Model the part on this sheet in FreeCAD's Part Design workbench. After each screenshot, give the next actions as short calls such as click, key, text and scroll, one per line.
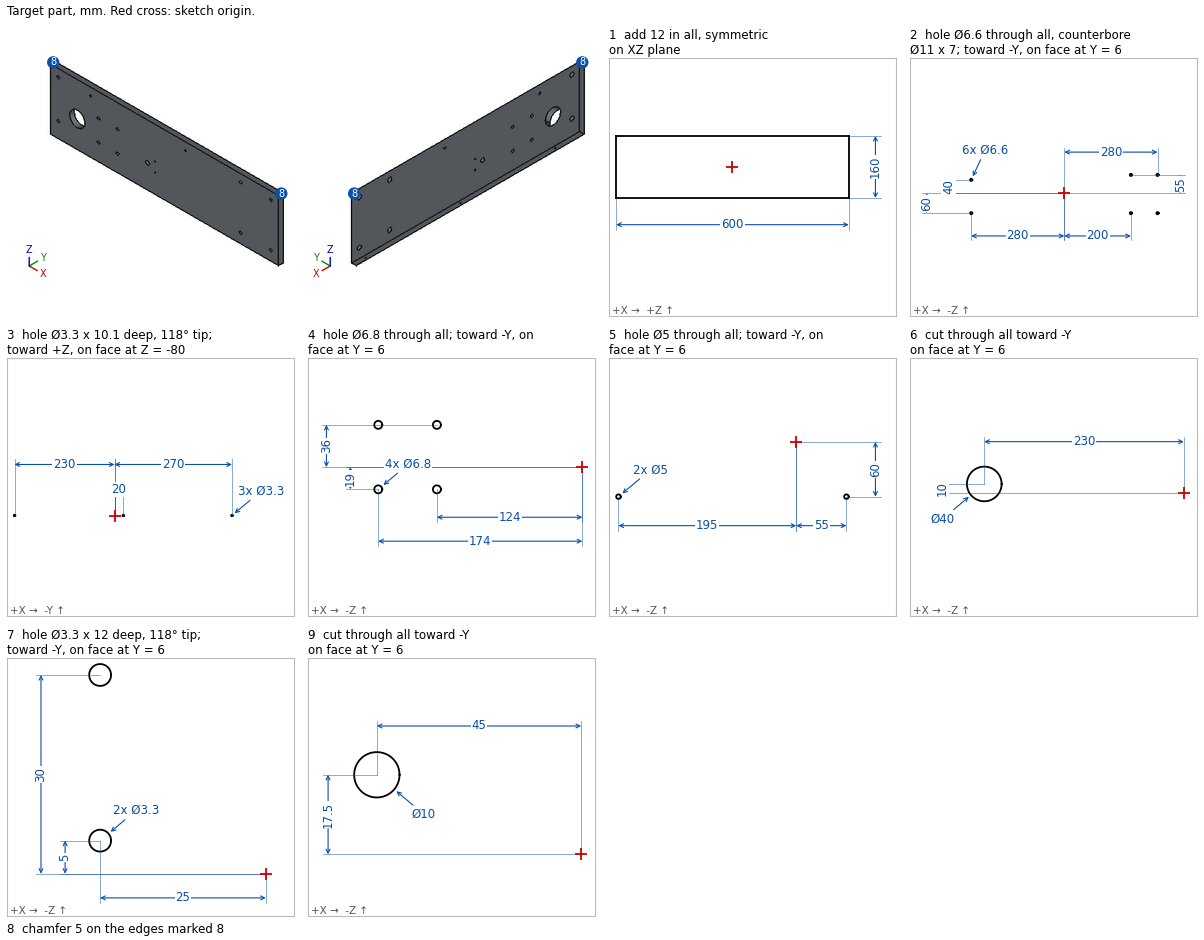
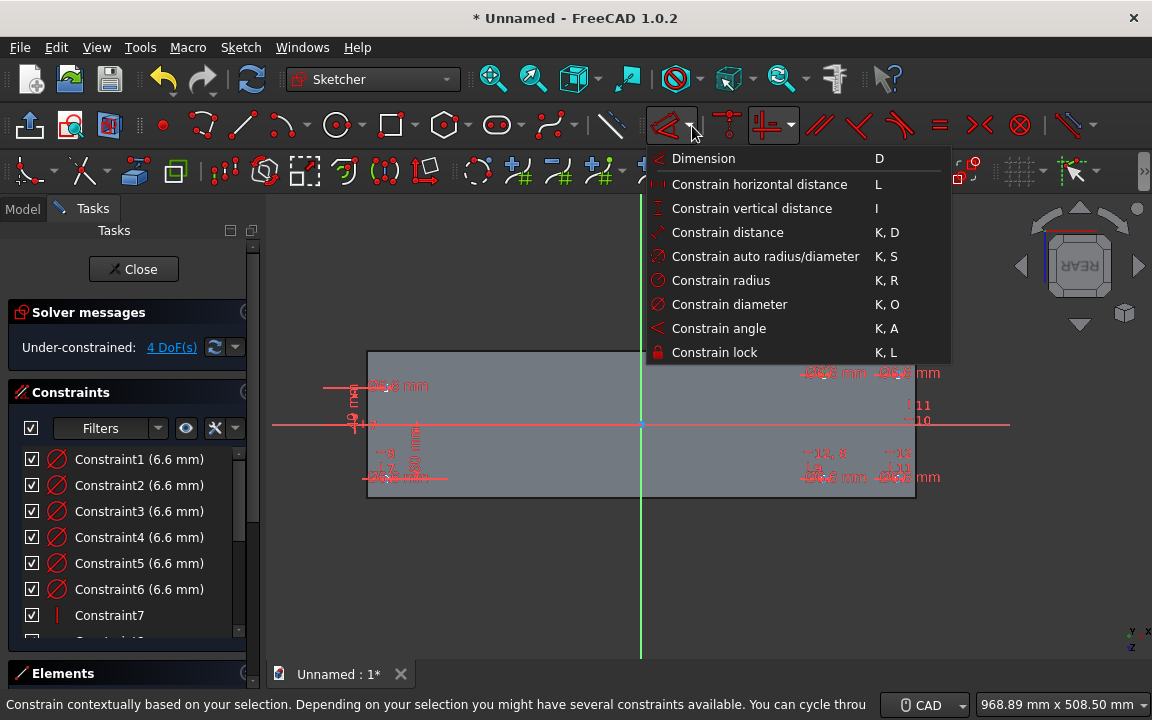
click(799, 208)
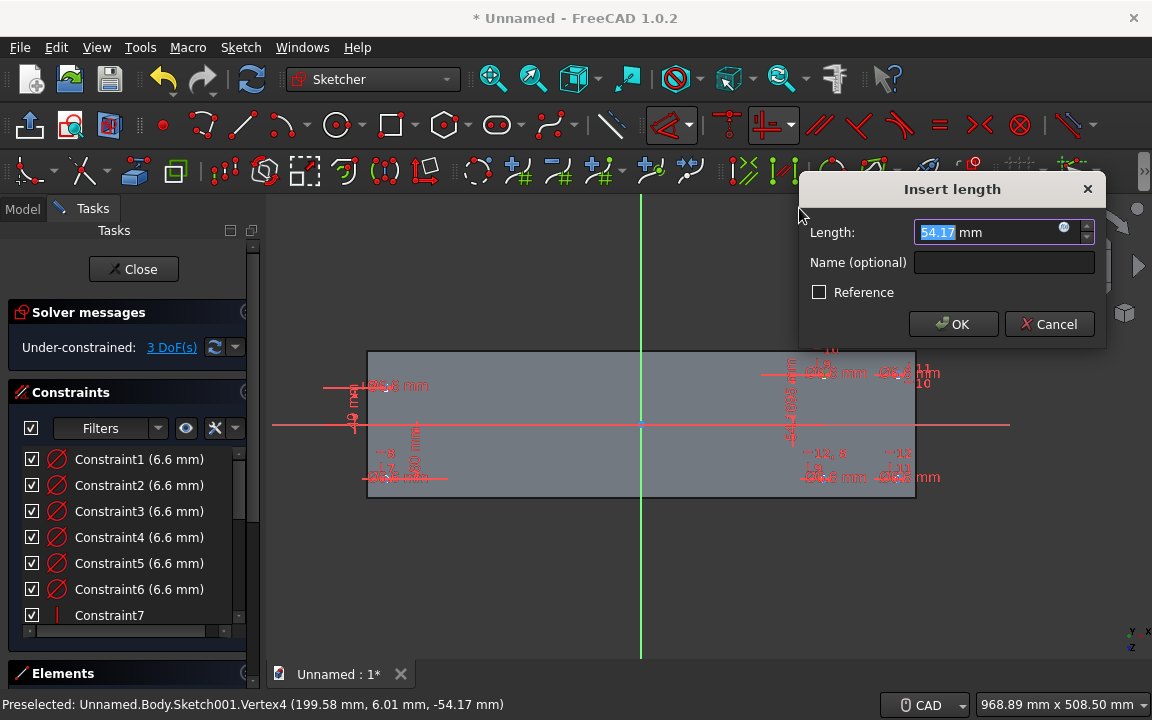
text(55)
key(Return)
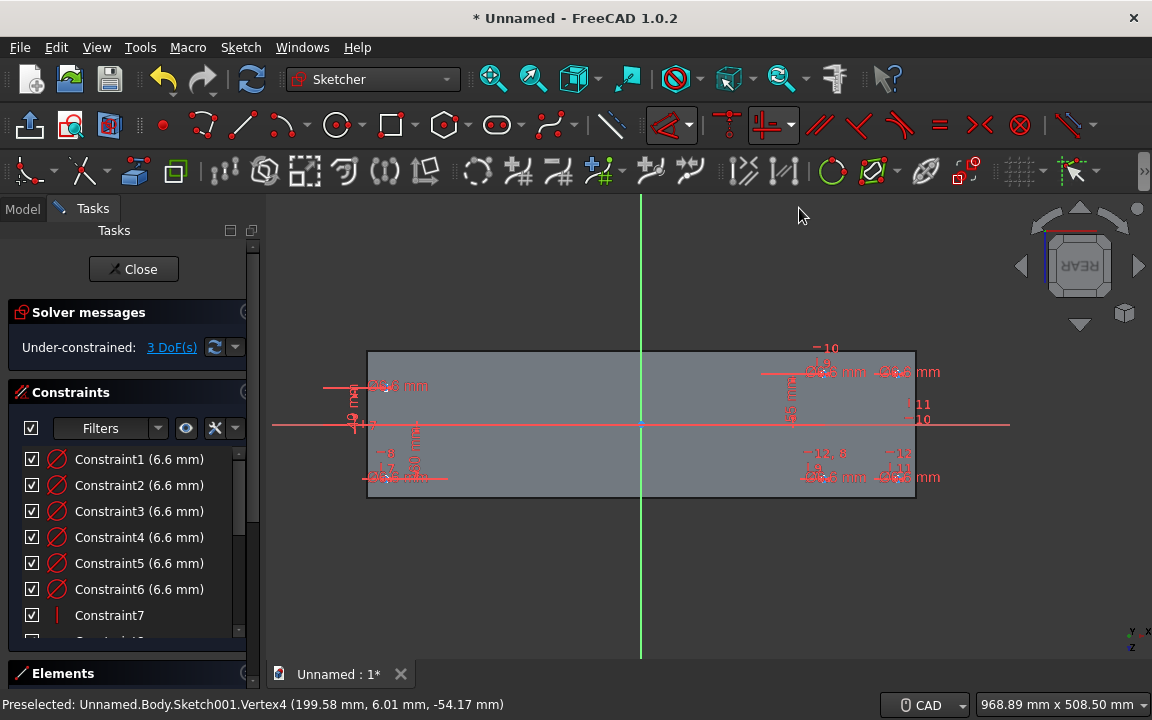
click(386, 479)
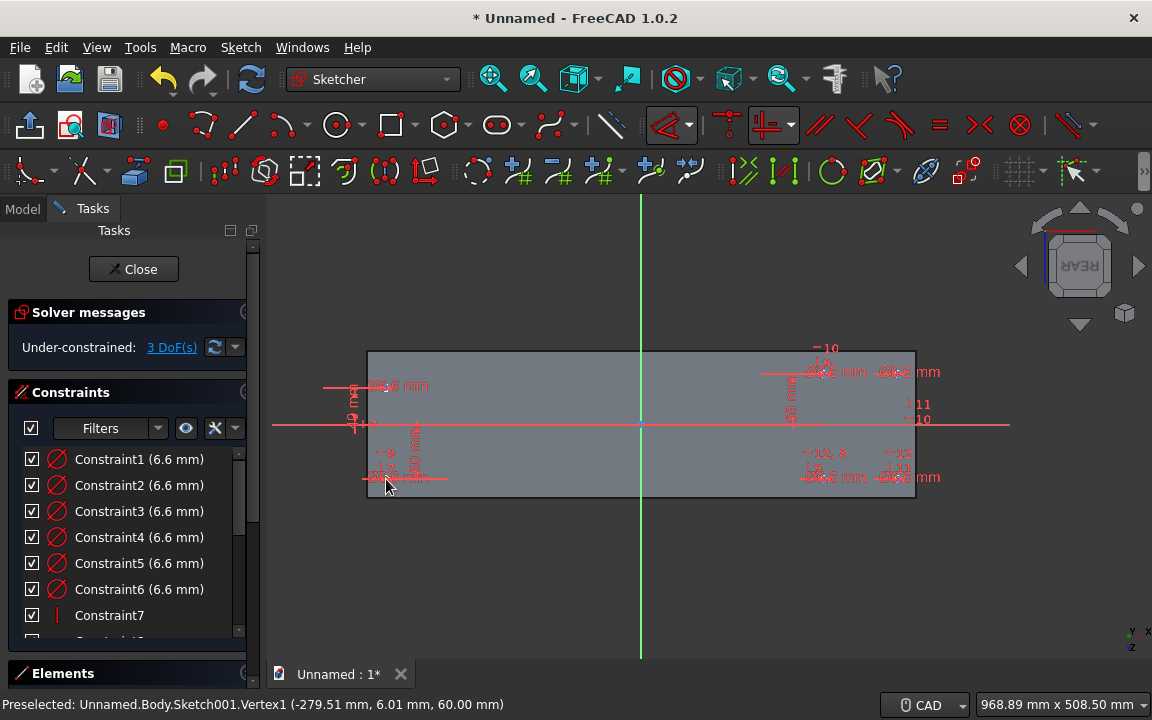
click(692, 126)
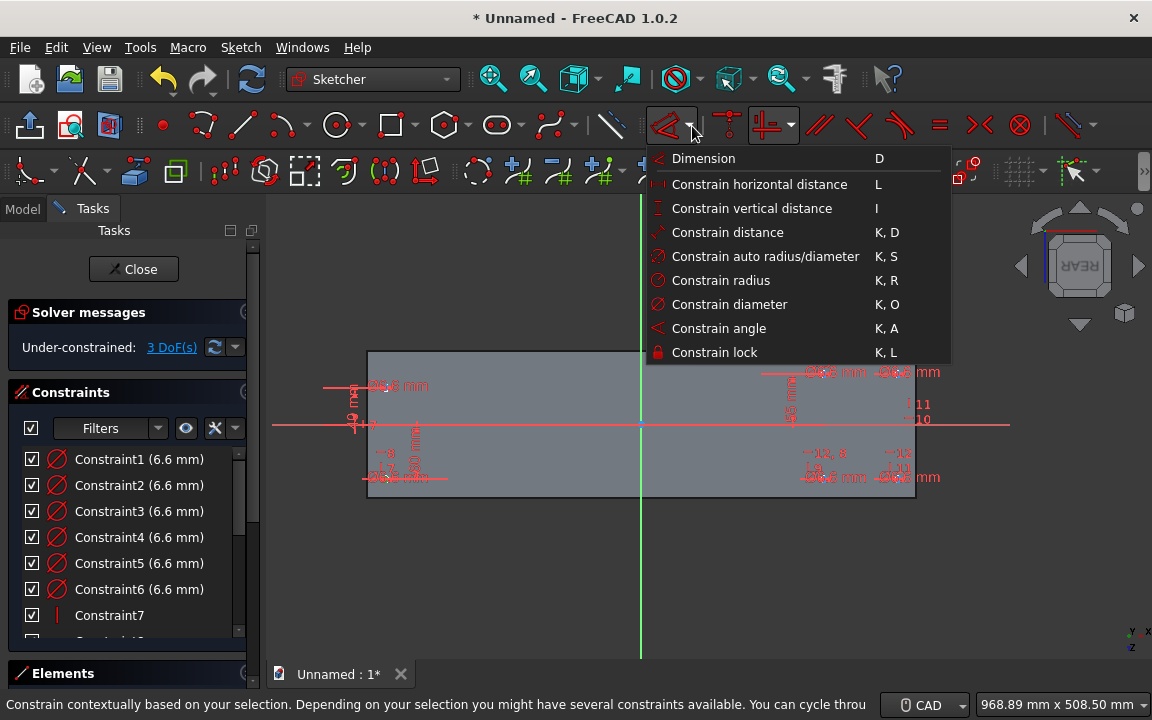
click(799, 184)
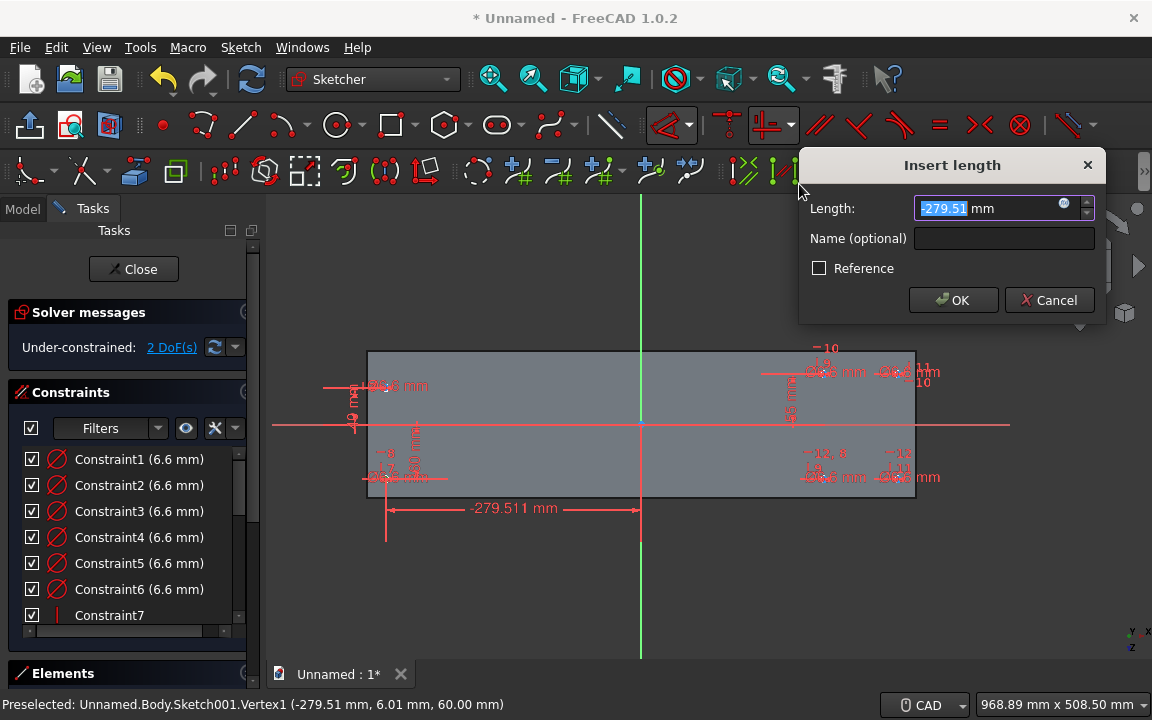
text(-280)
key(Return)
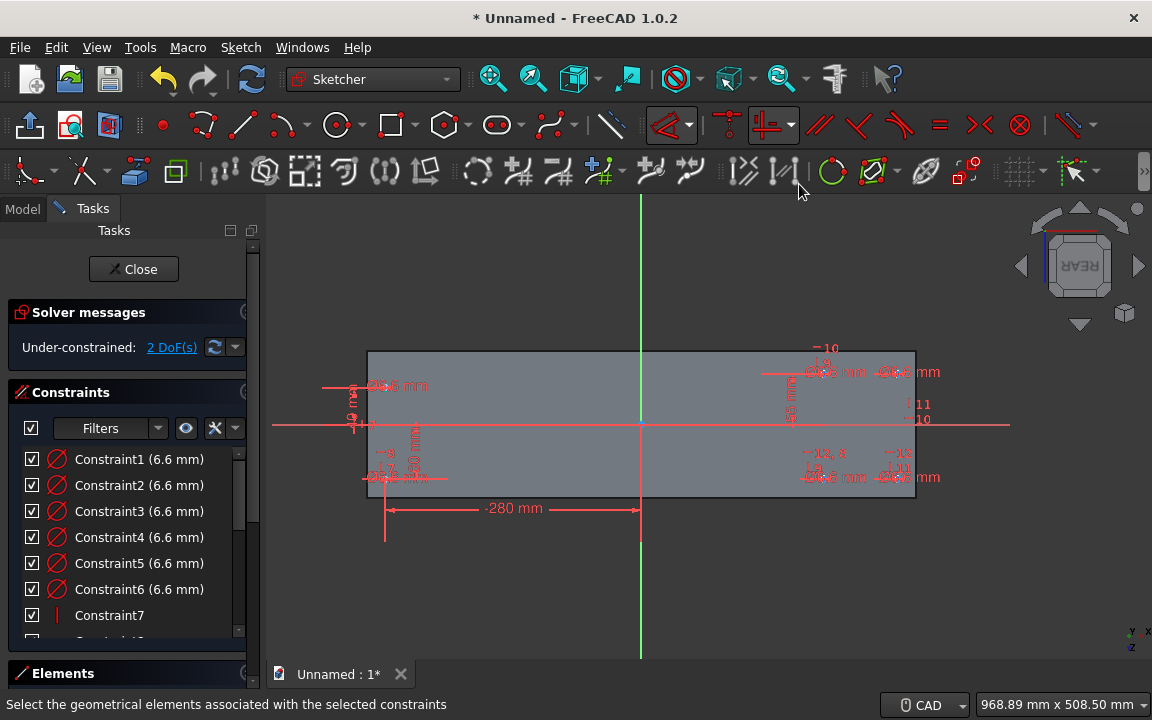
click(824, 479)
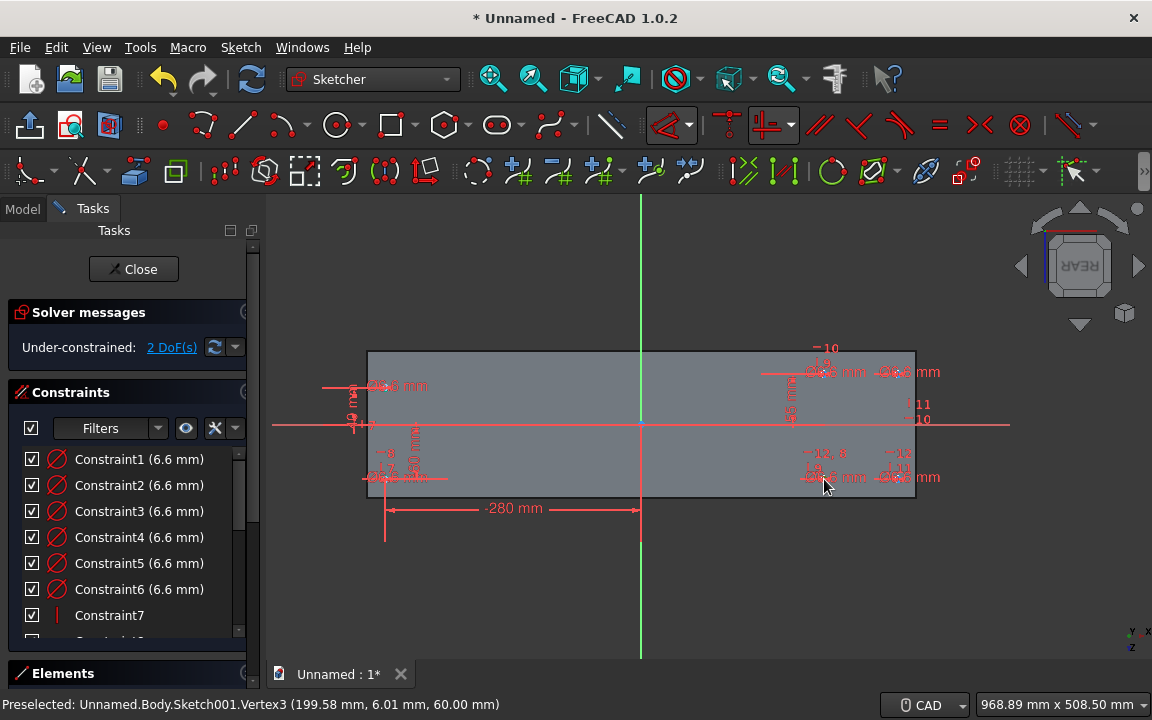
click(692, 126)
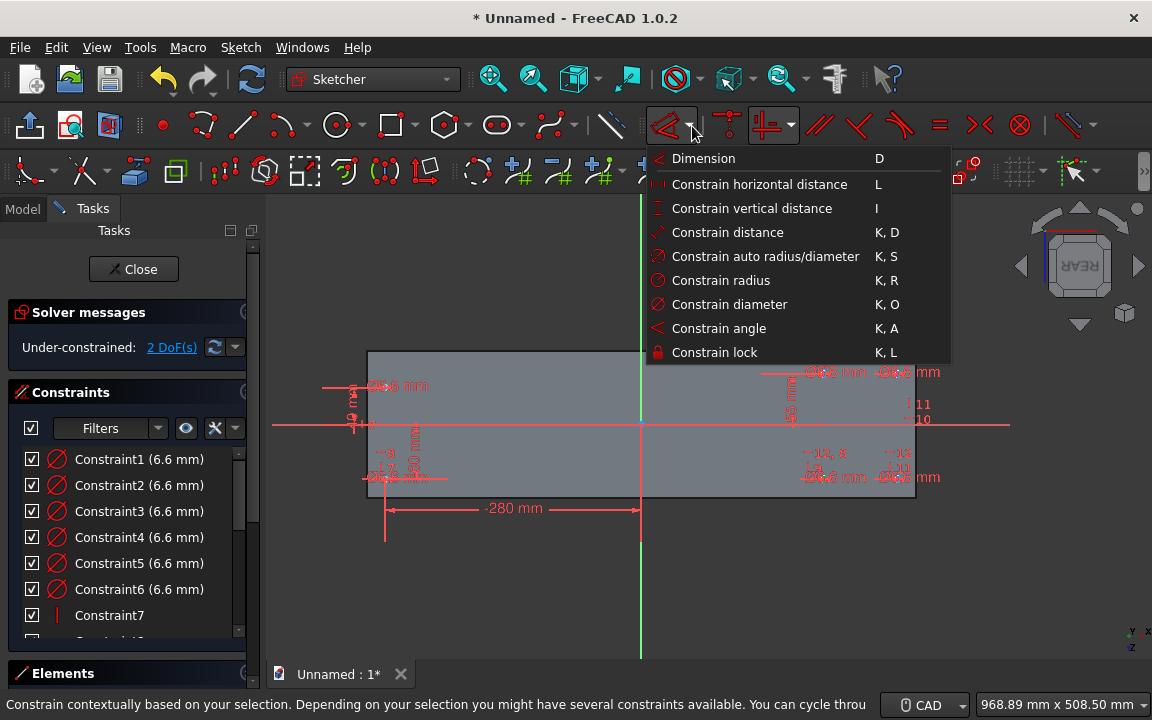
click(799, 184)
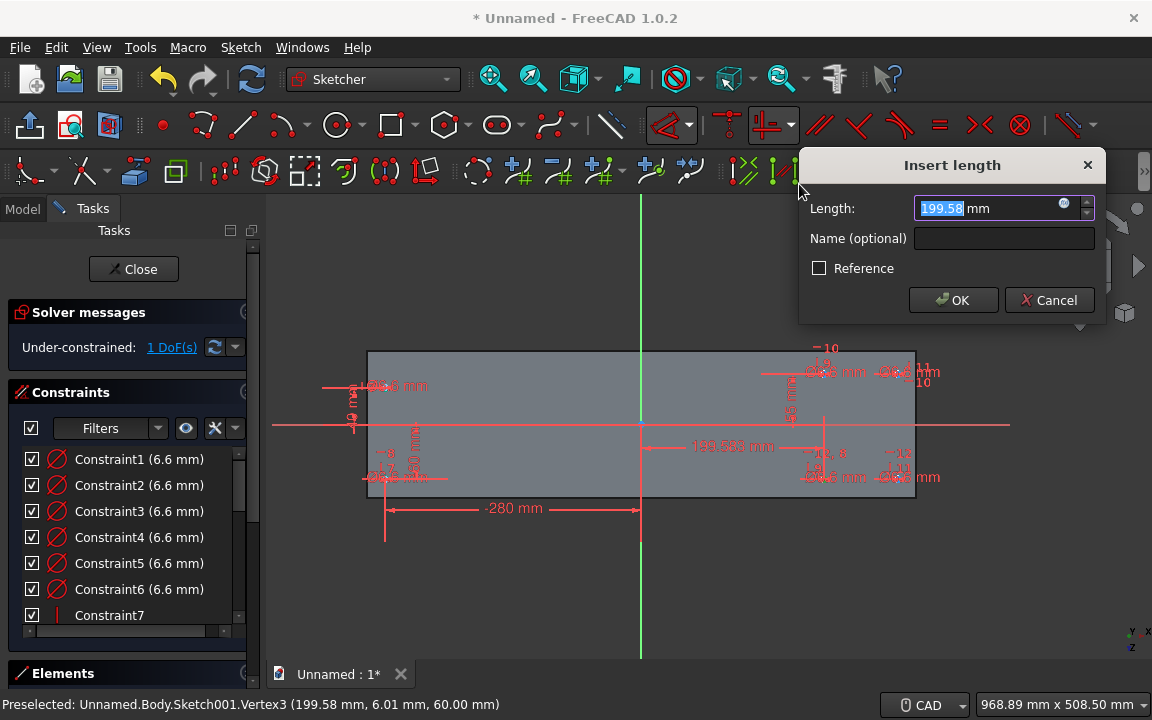
text(200)
key(Return)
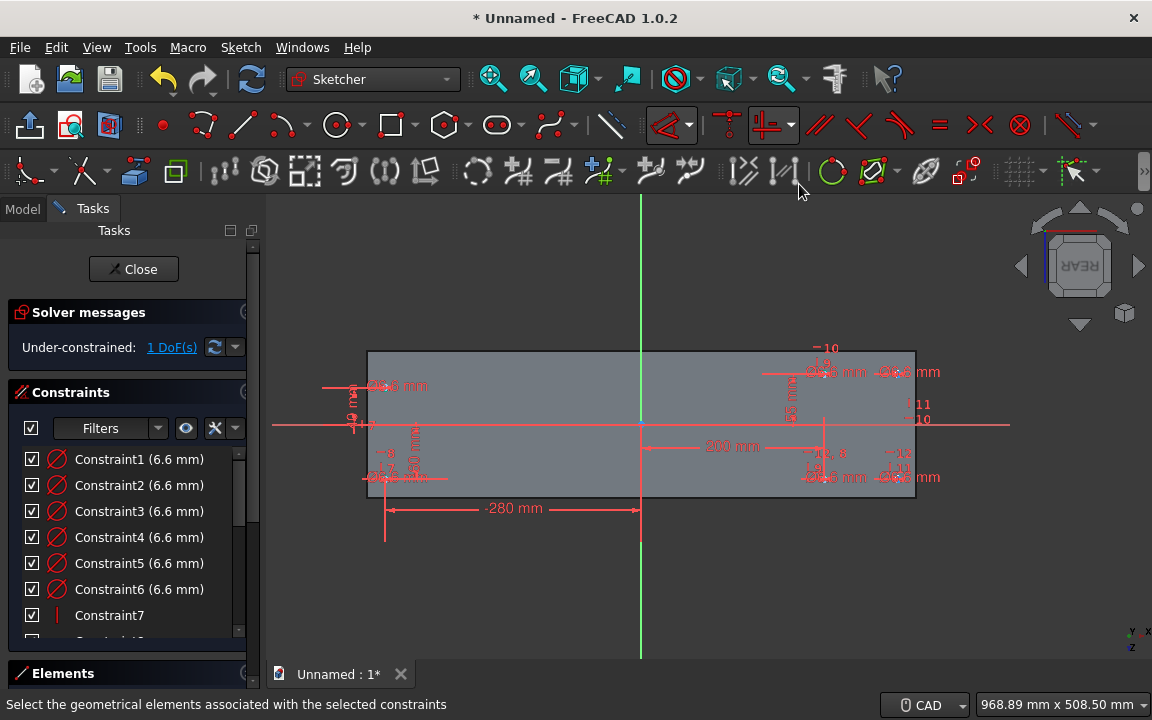
click(898, 374)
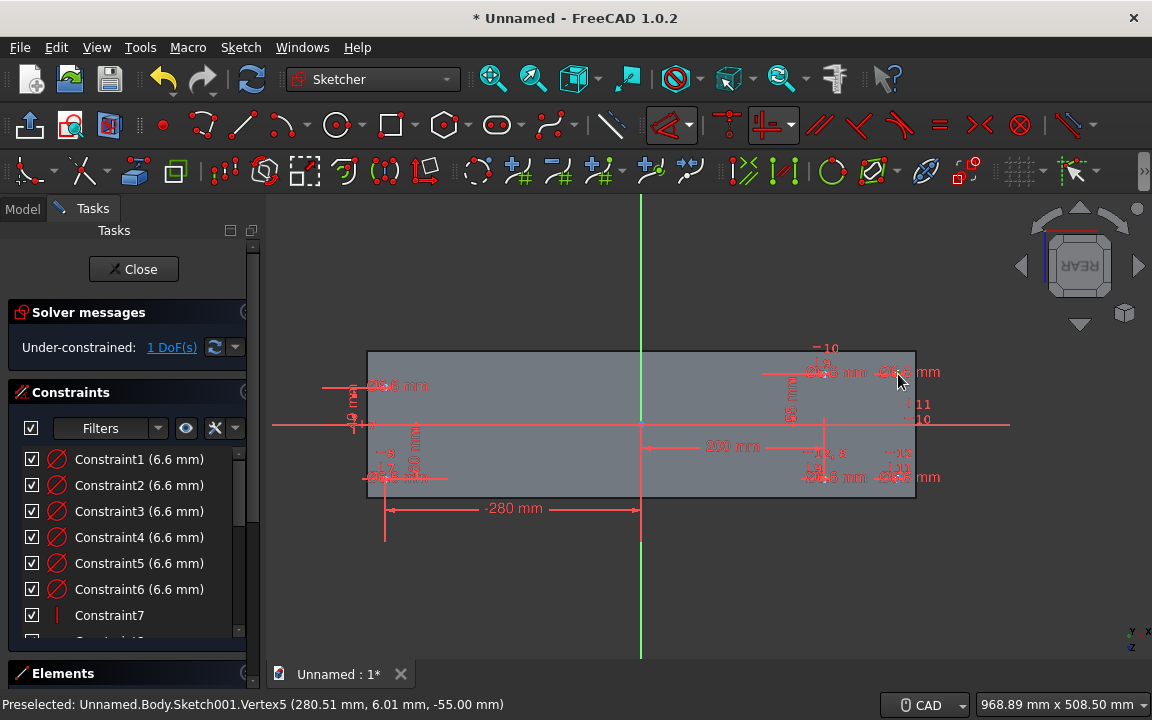
key(l)